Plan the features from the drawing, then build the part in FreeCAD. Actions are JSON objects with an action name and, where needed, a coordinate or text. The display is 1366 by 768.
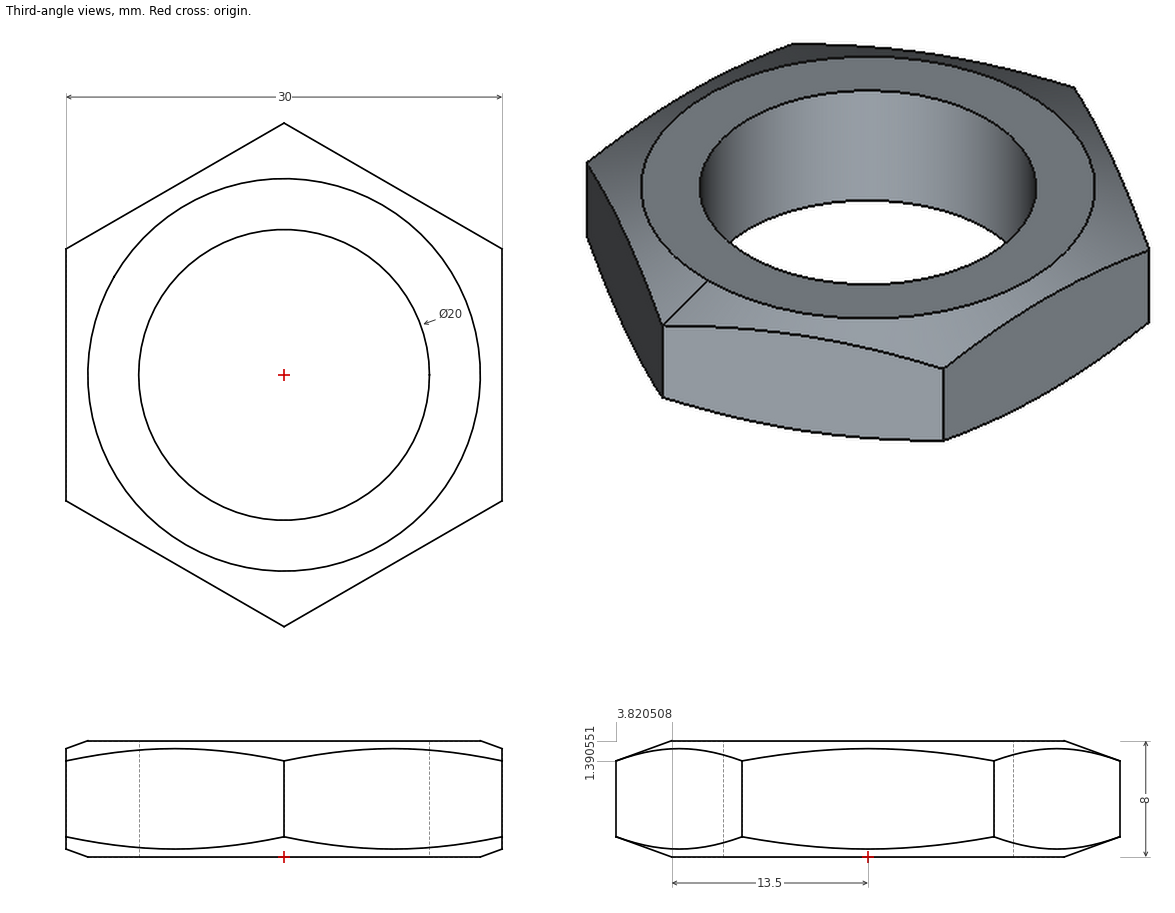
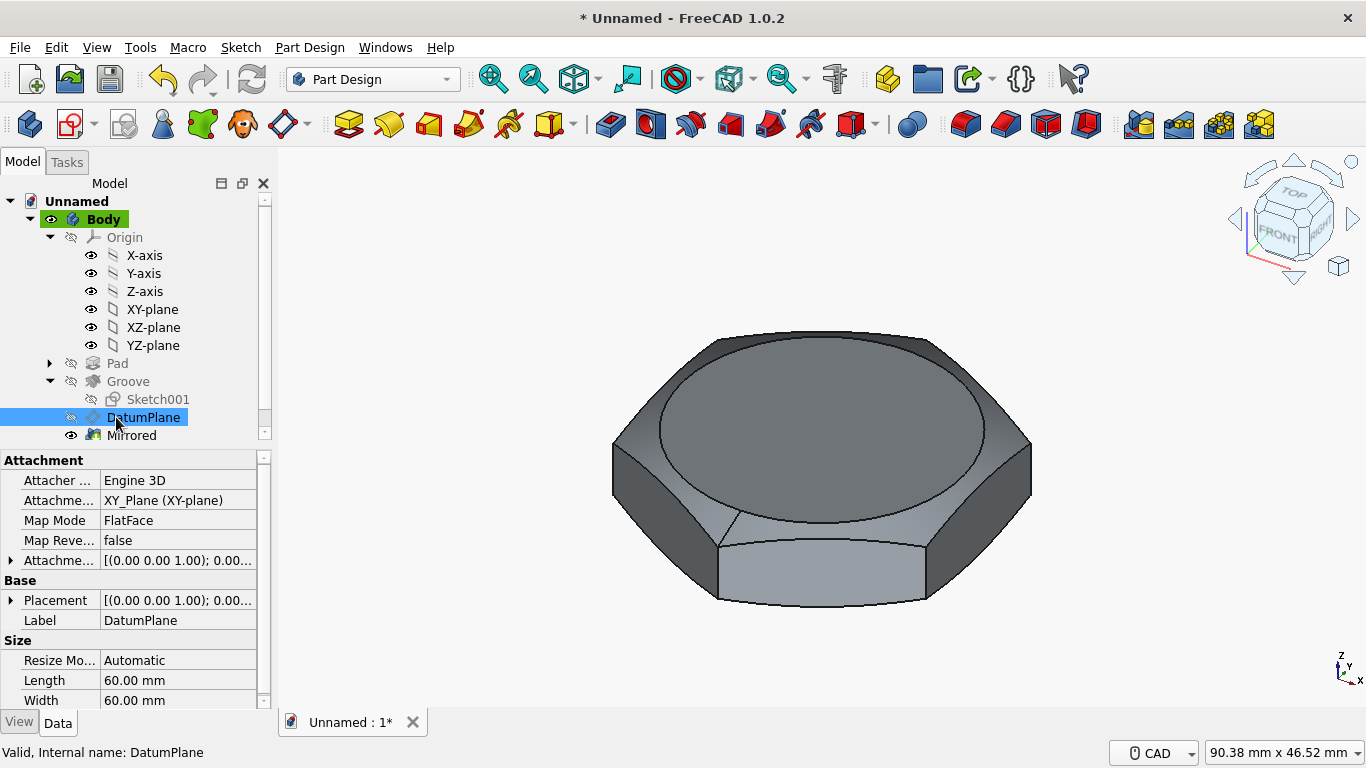
{"action": "left_click", "coordinate": [822, 429]}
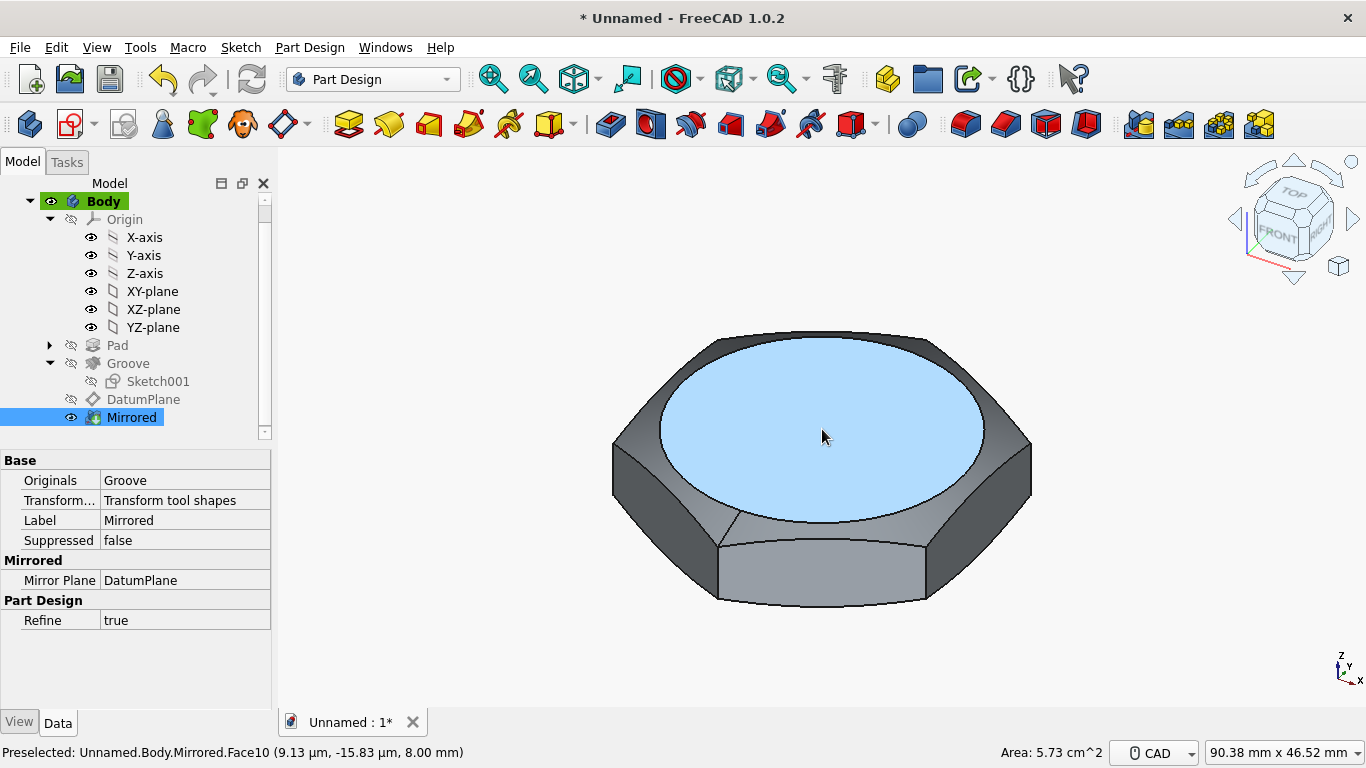
{"action": "left_click", "coordinate": [70, 124]}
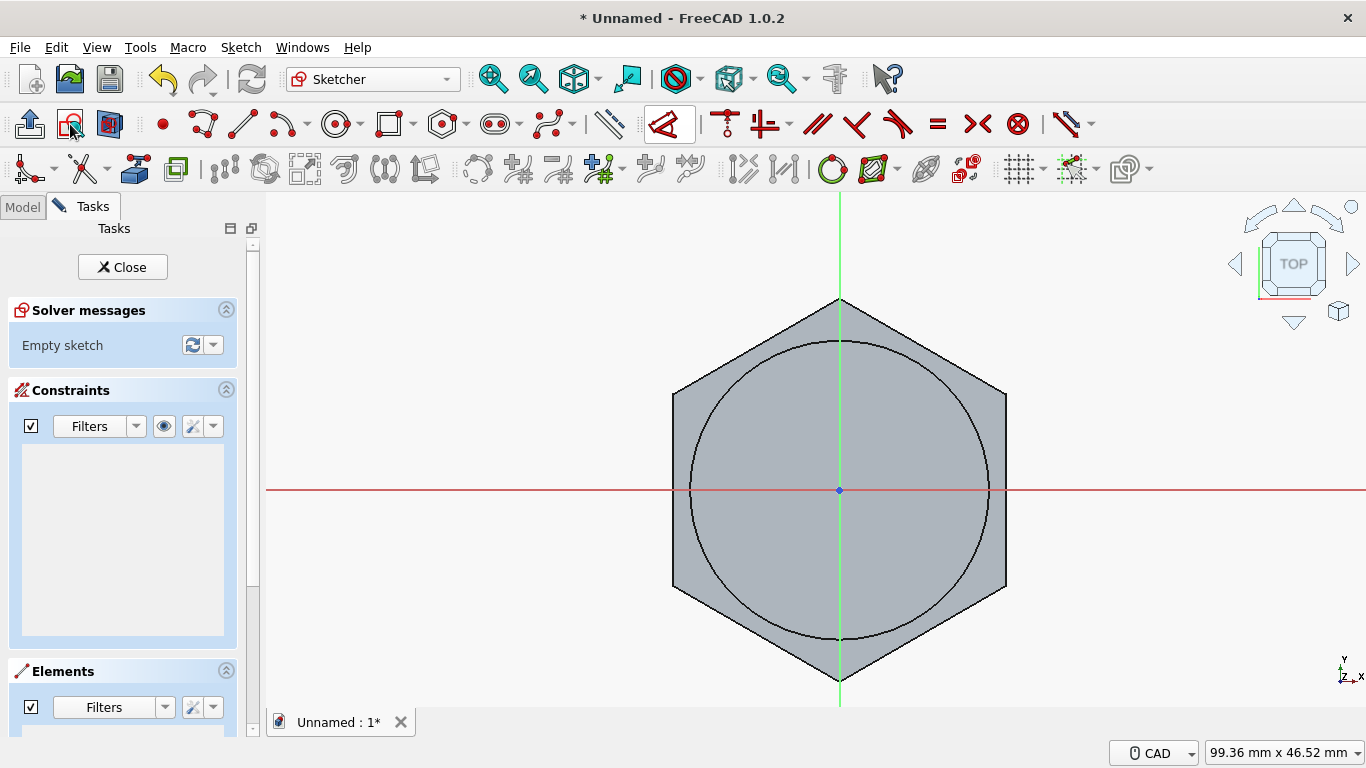
{"action": "scroll", "coordinate": [1027, 573], "scroll_direction": "up", "scroll_amount": 2}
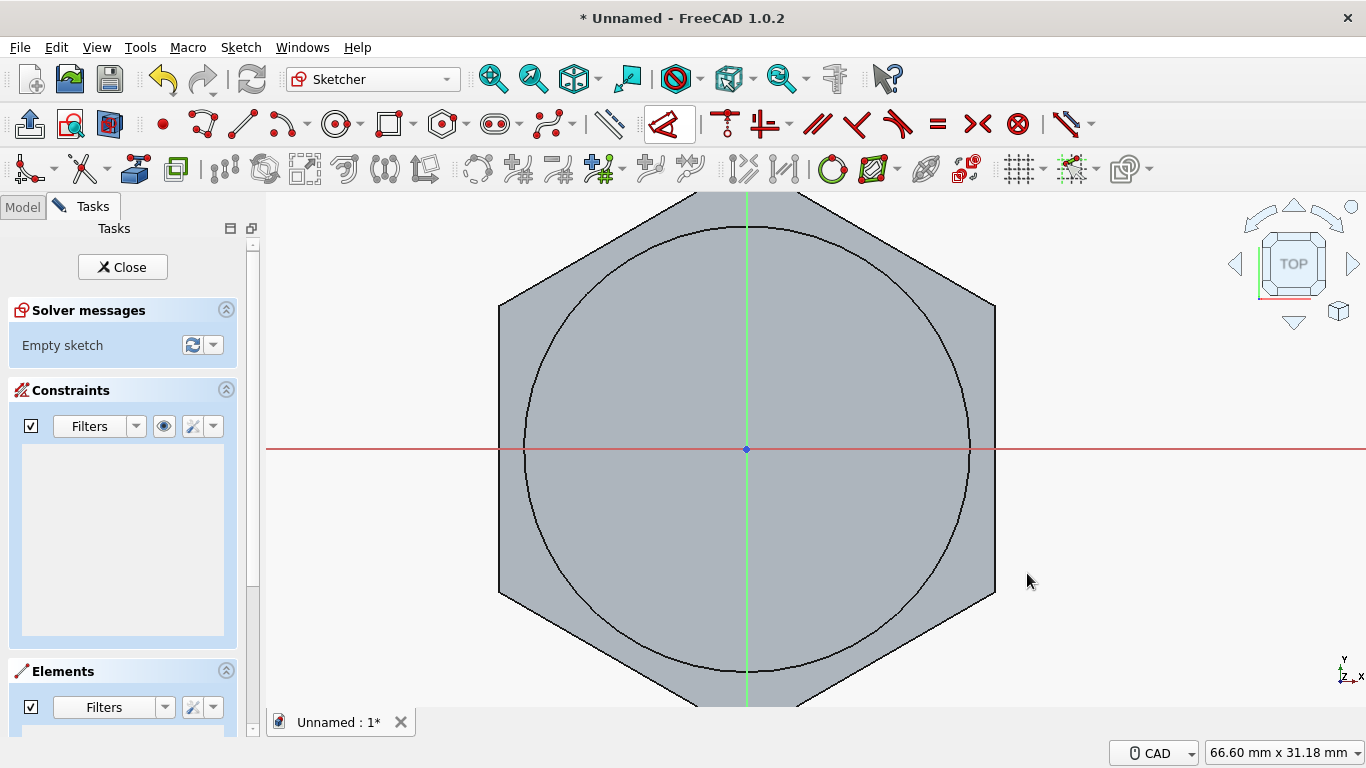
{"action": "key", "text": "g c"}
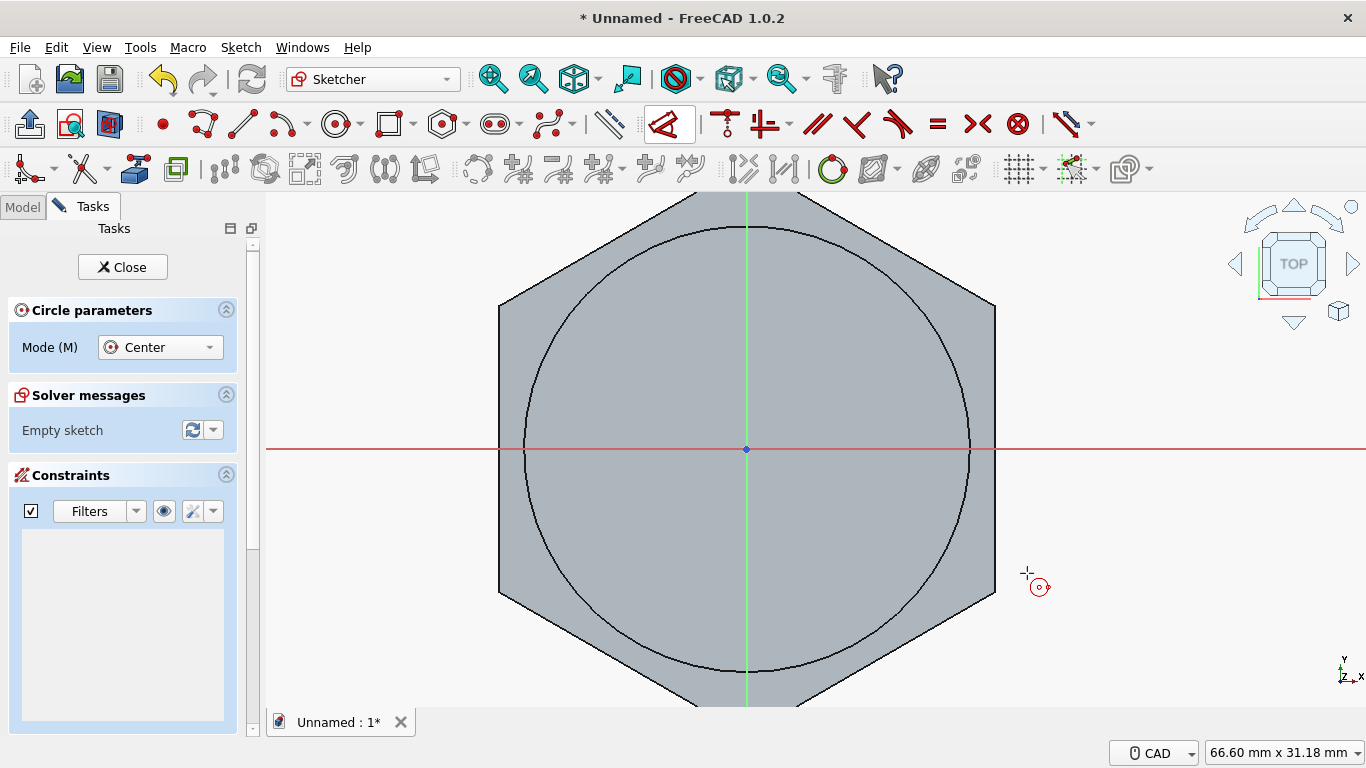
{"action": "left_click", "coordinate": [747, 449]}
{"action": "left_click", "coordinate": [864, 332]}
{"action": "key", "text": "Escape"}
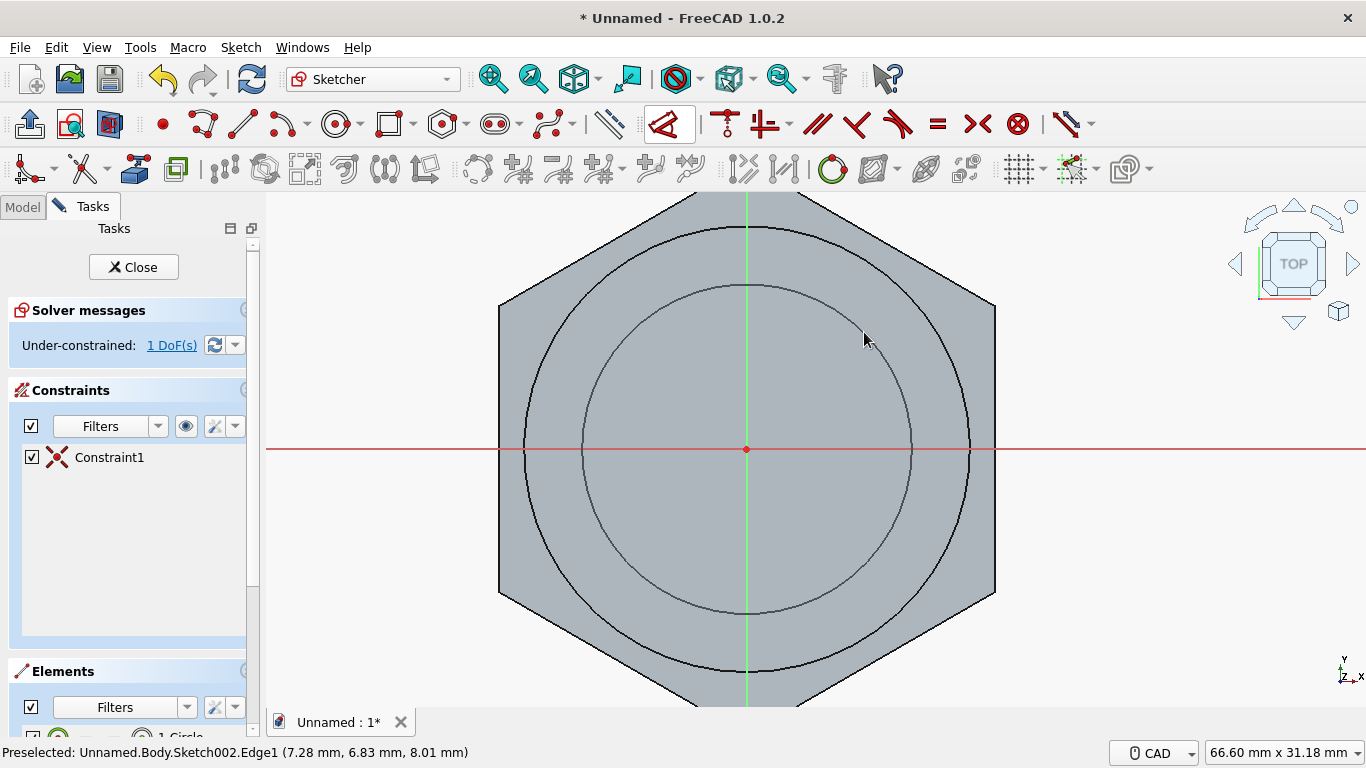
{"action": "key", "text": "d"}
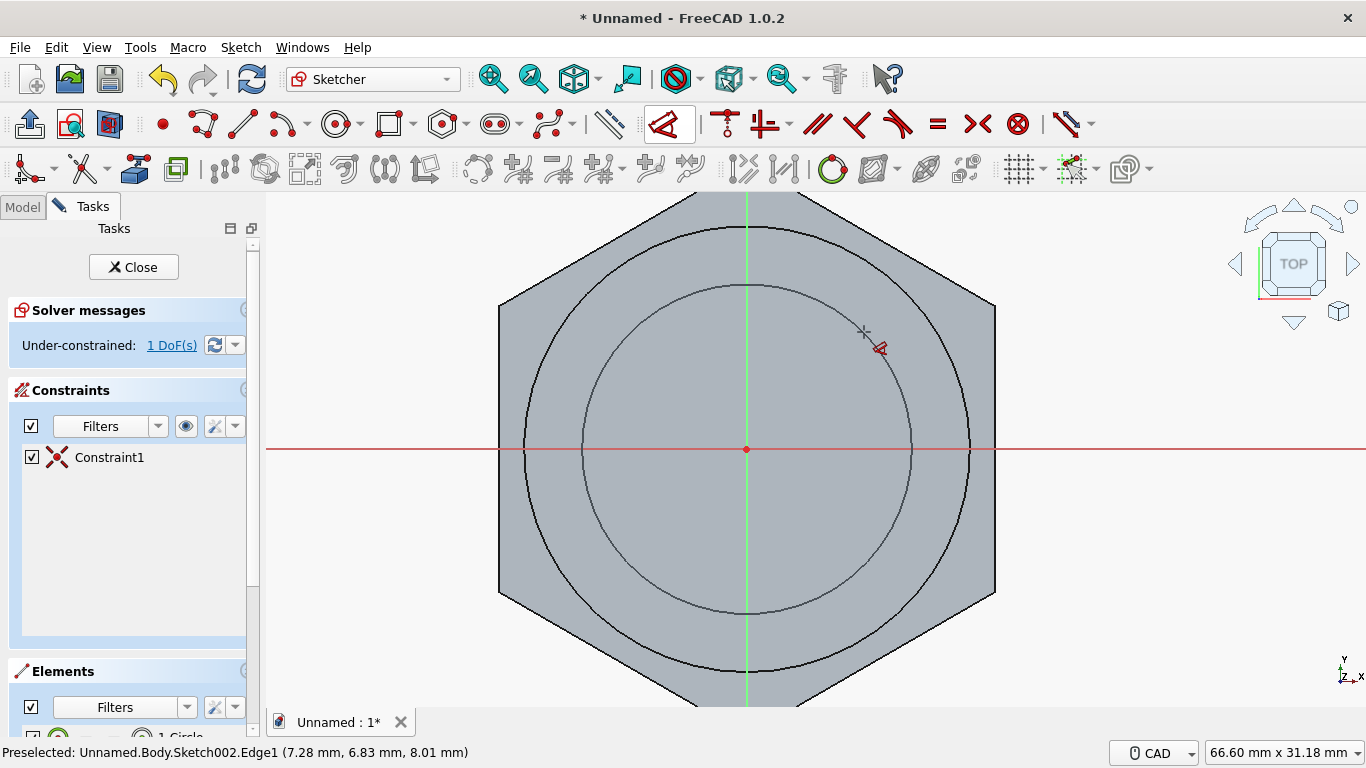
{"action": "left_click", "coordinate": [863, 332]}
{"action": "left_click", "coordinate": [886, 309]}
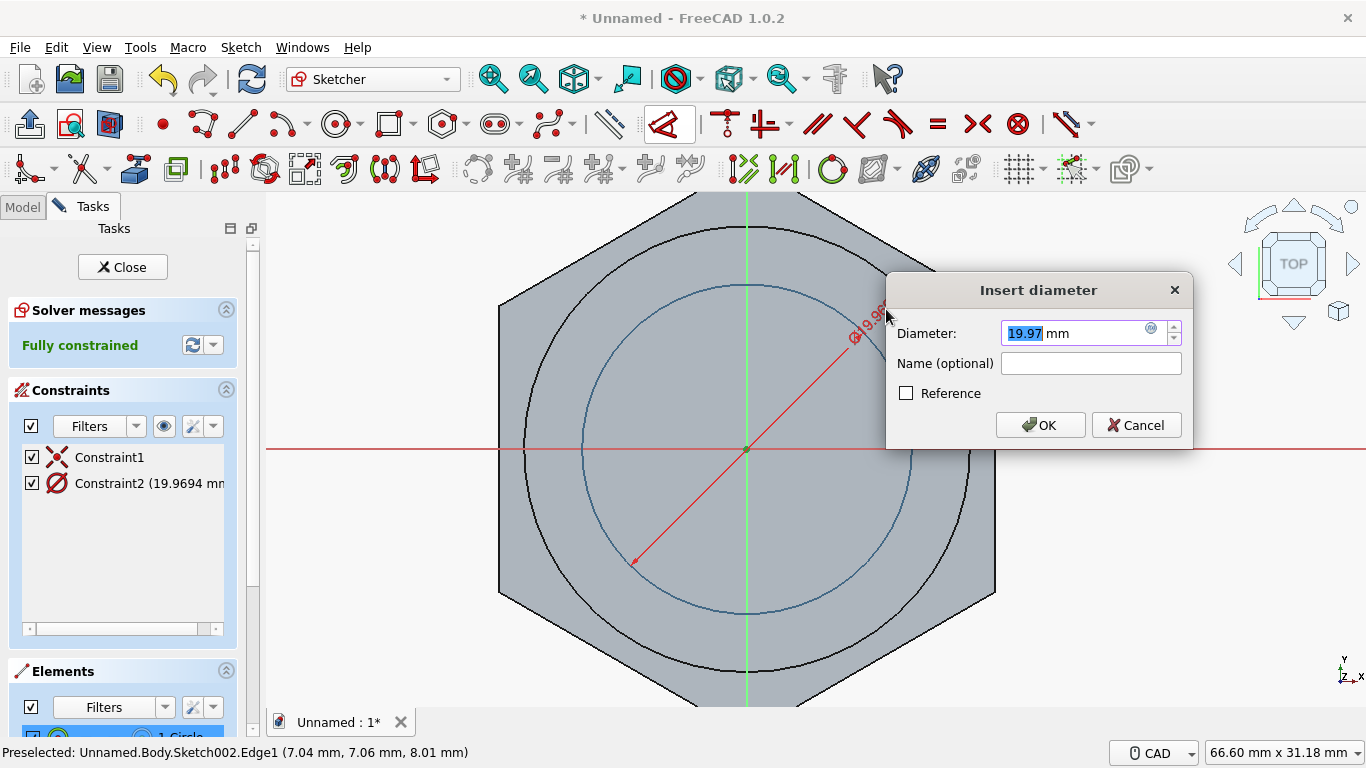
{"action": "type", "text": "20"}
{"action": "key", "text": "Return"}
{"action": "key", "text": "Escape"}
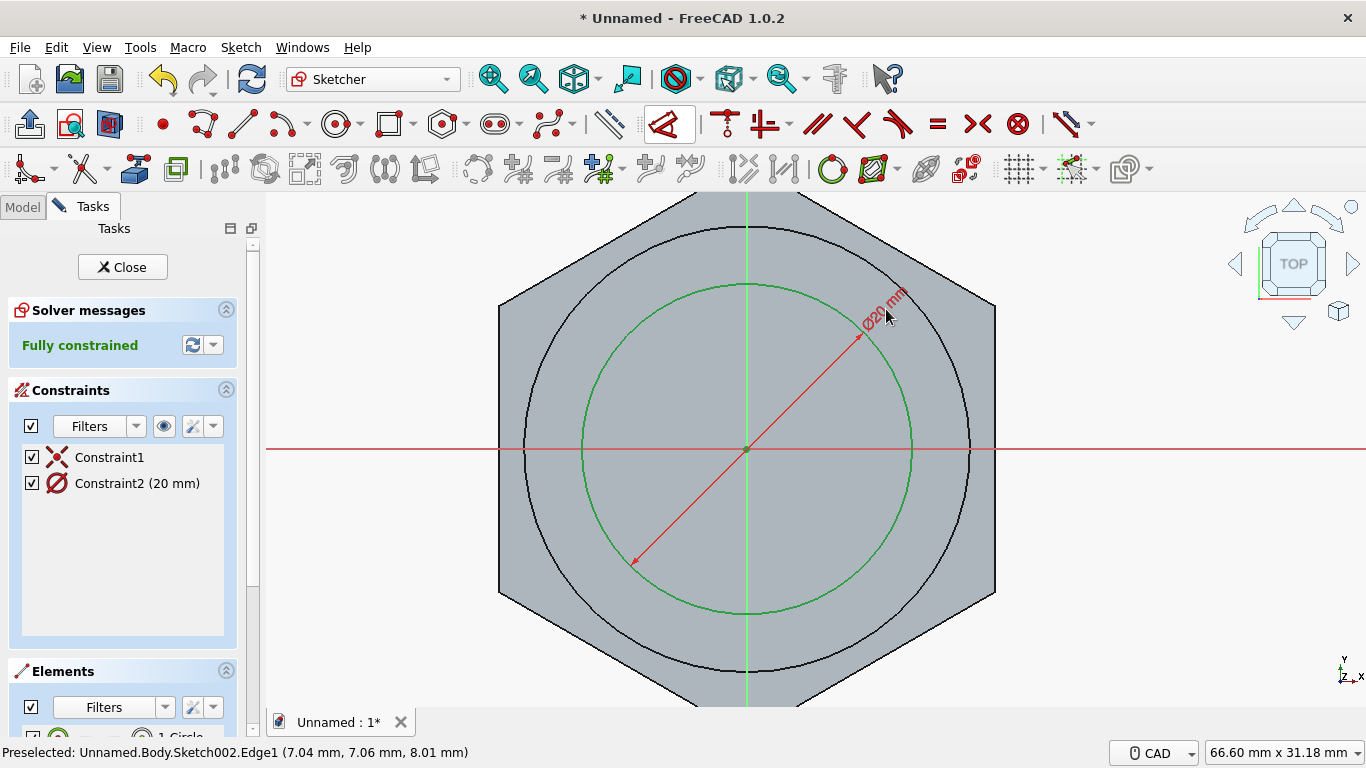
{"action": "left_click", "coordinate": [123, 267]}